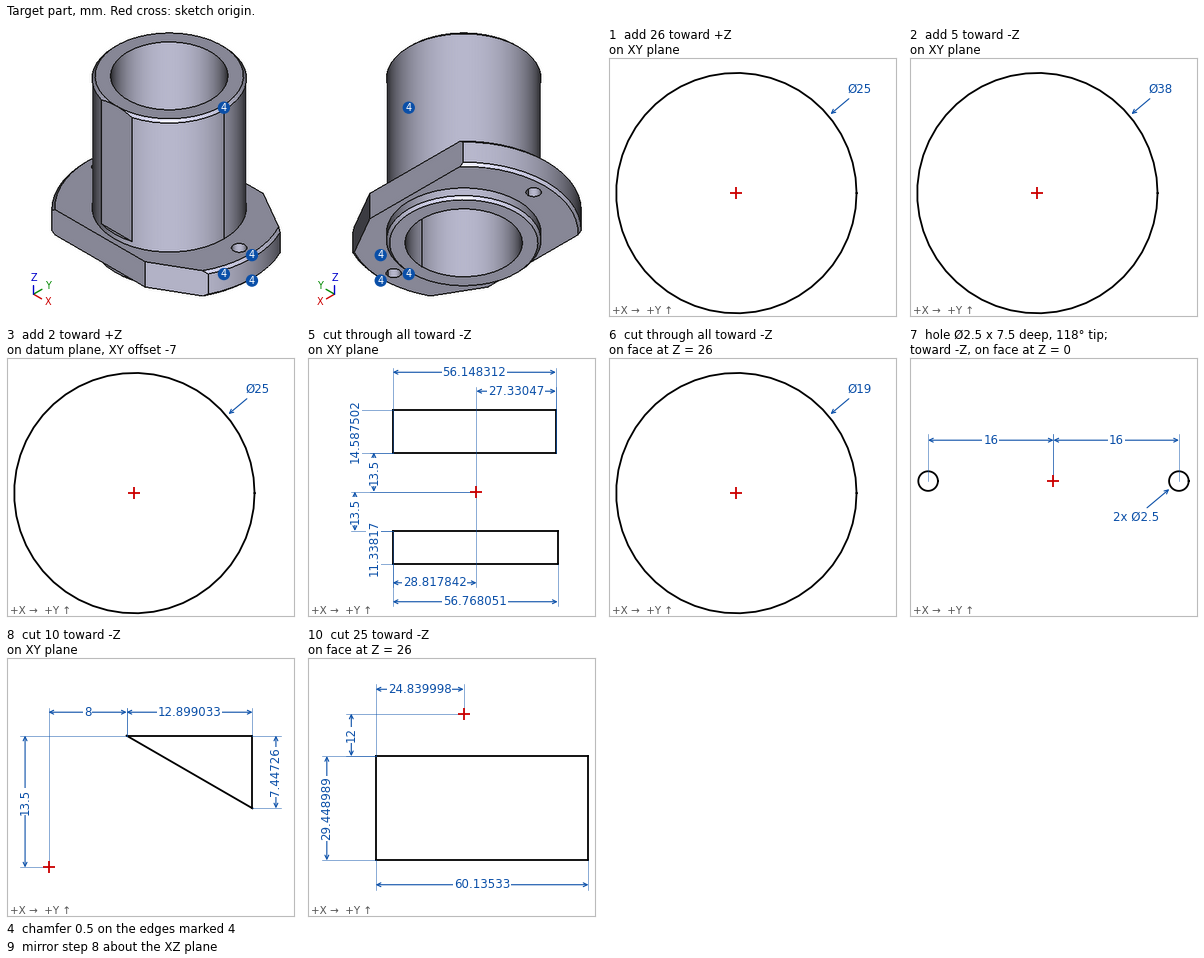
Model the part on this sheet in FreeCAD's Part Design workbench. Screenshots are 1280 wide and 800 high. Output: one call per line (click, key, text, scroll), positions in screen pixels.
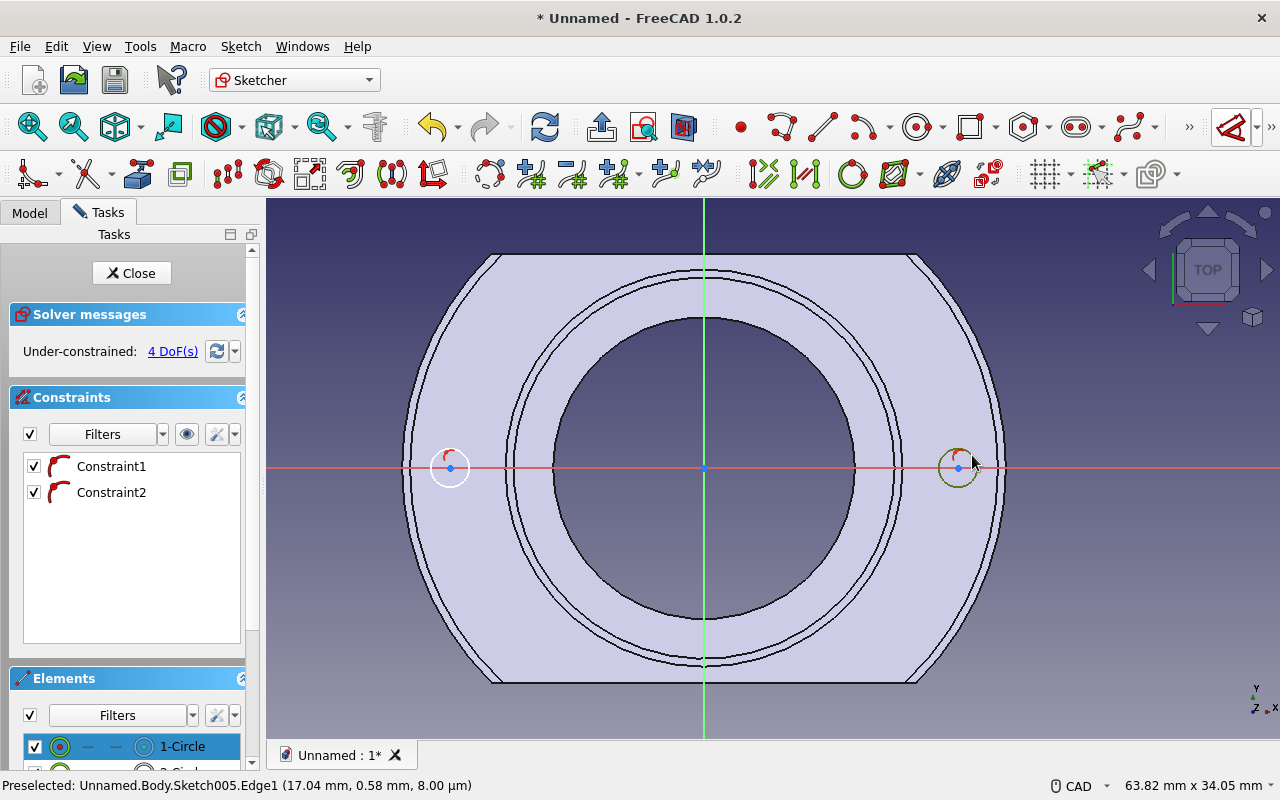
click(464, 455)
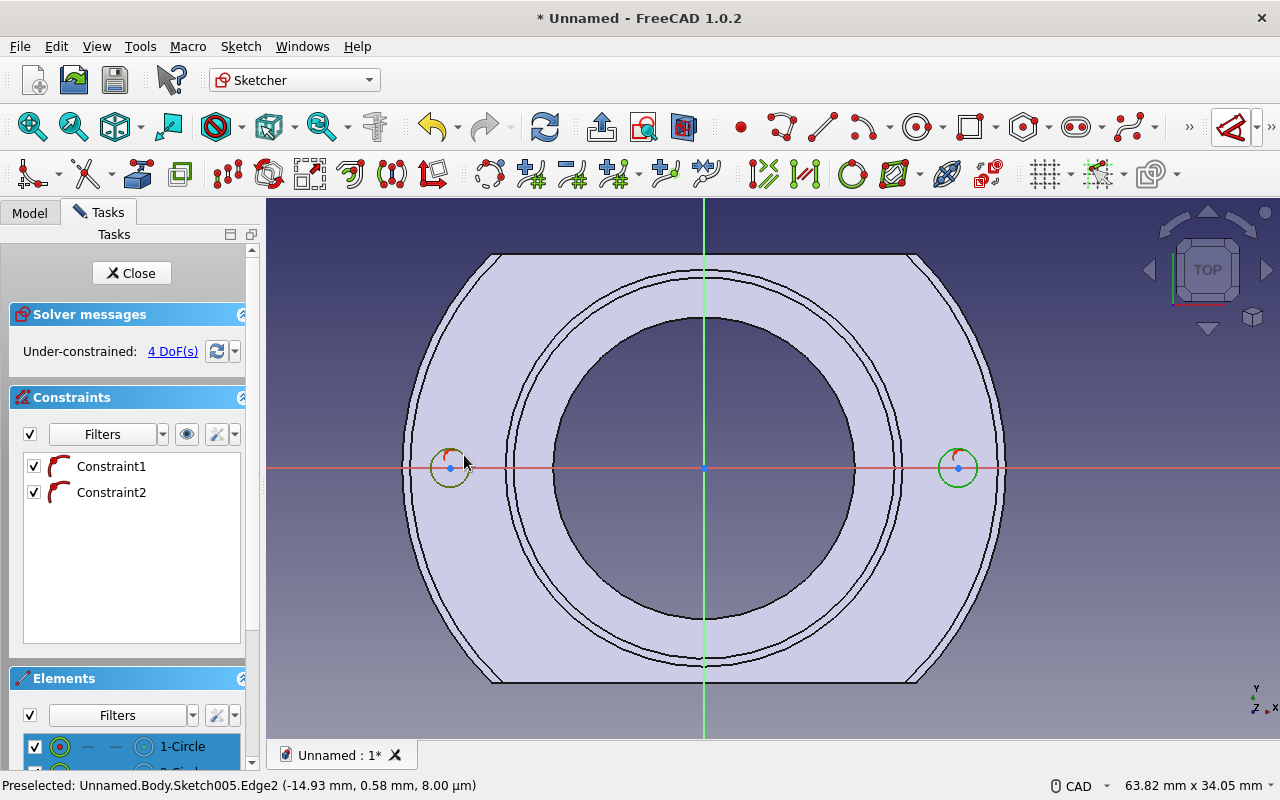
key(e)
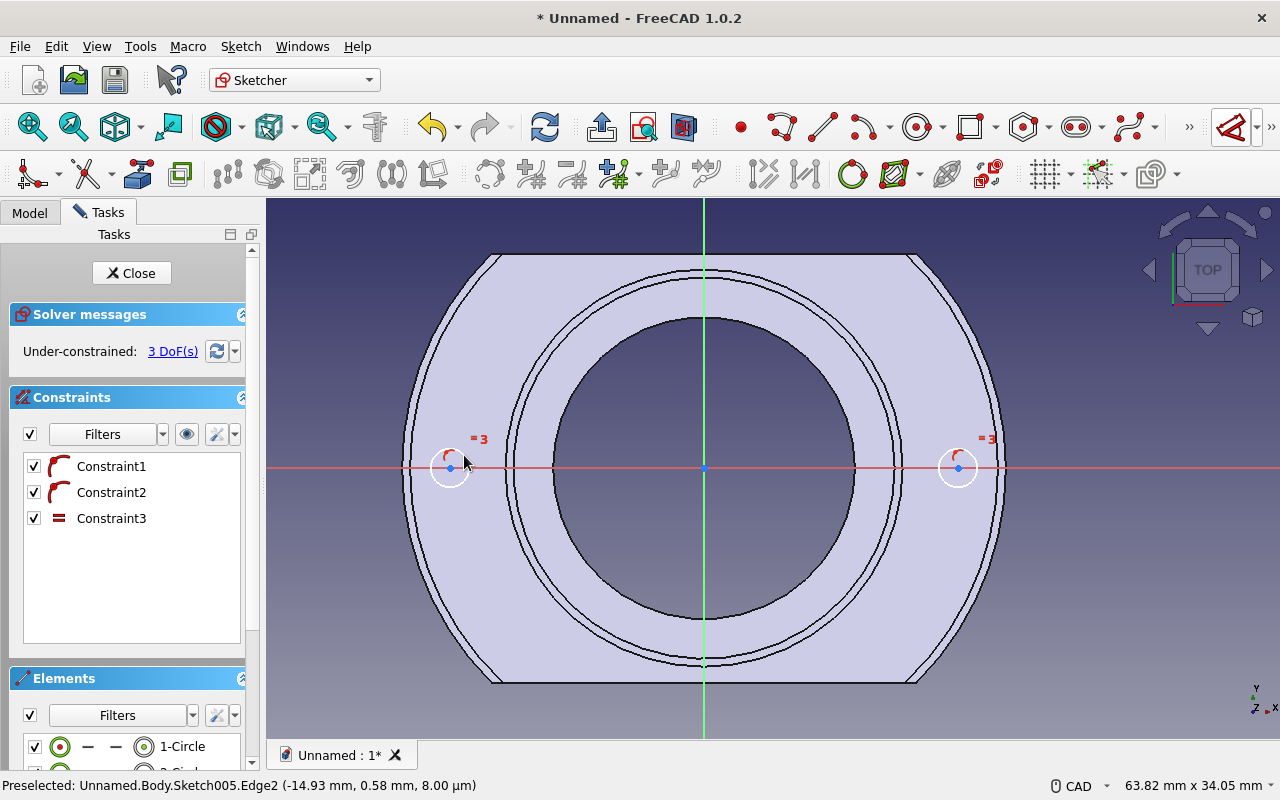
click(972, 455)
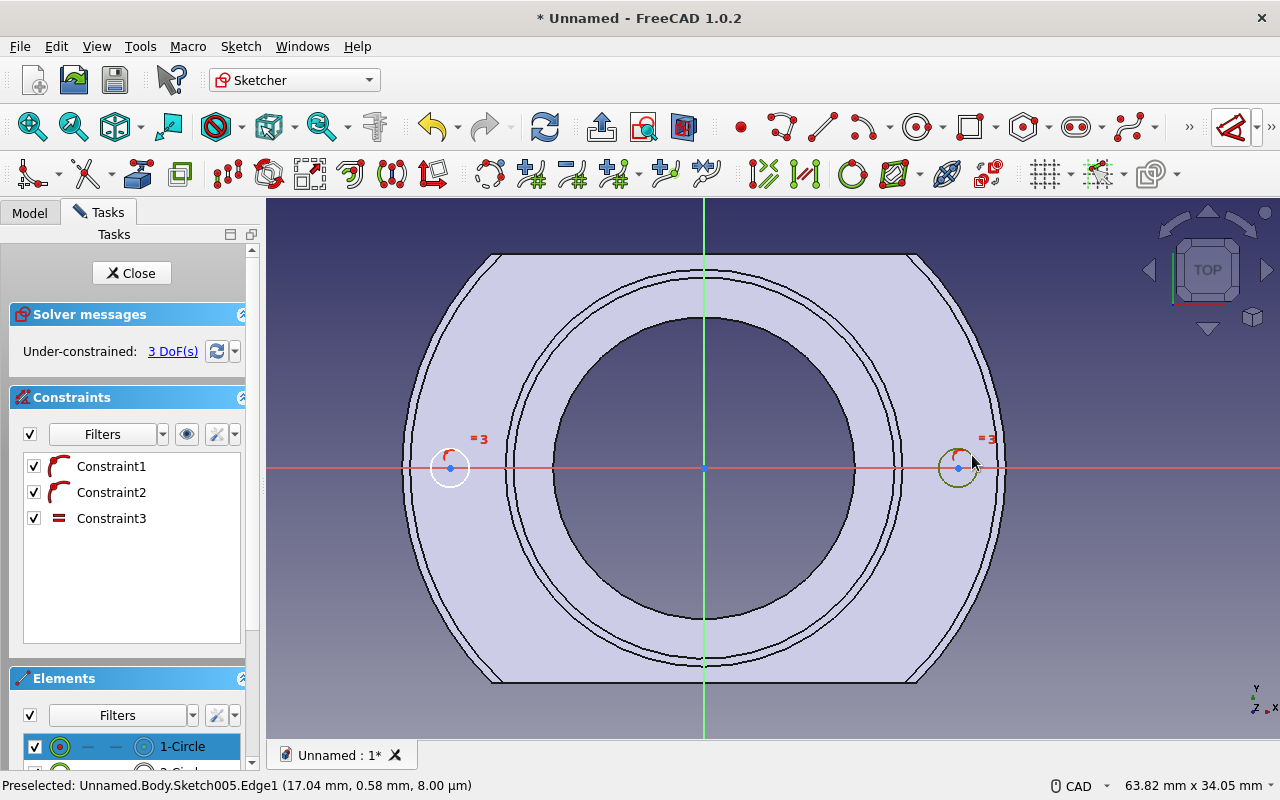
key(k)
key(o)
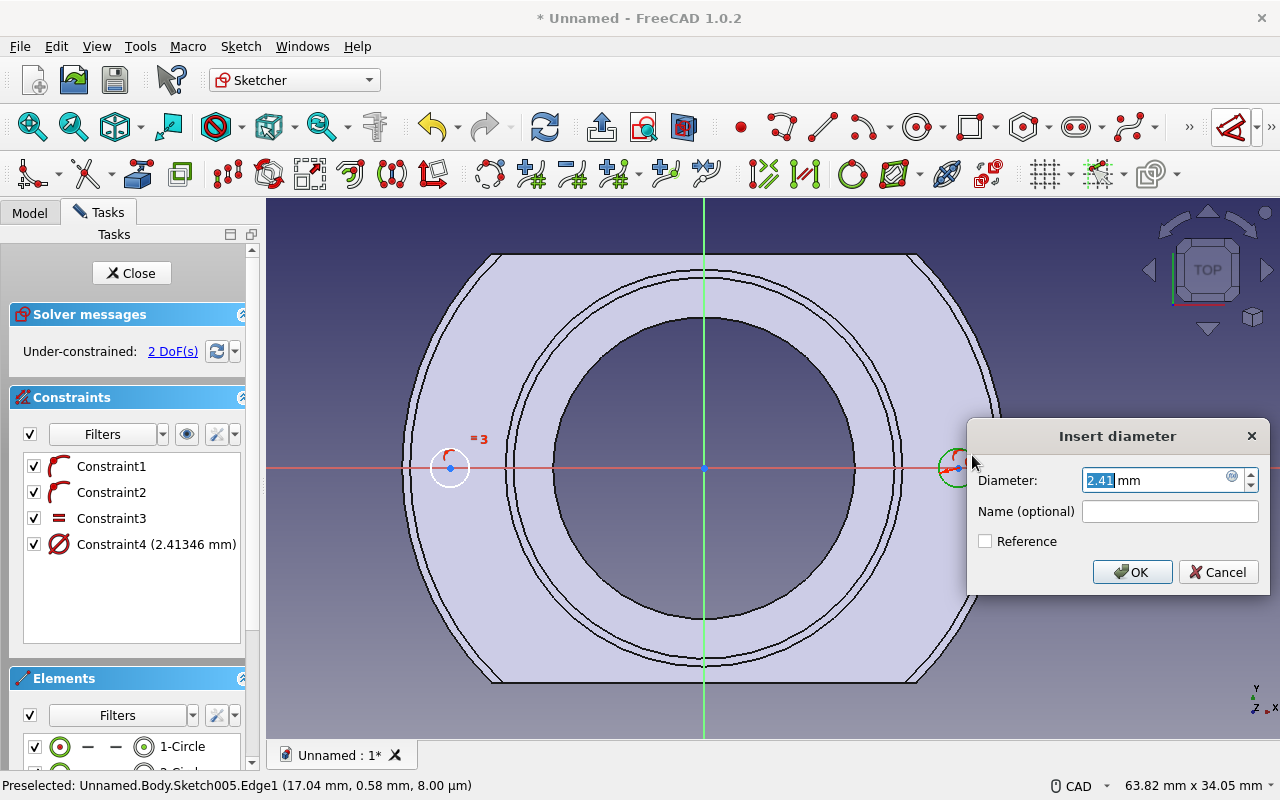
text(2.5)
key(Return)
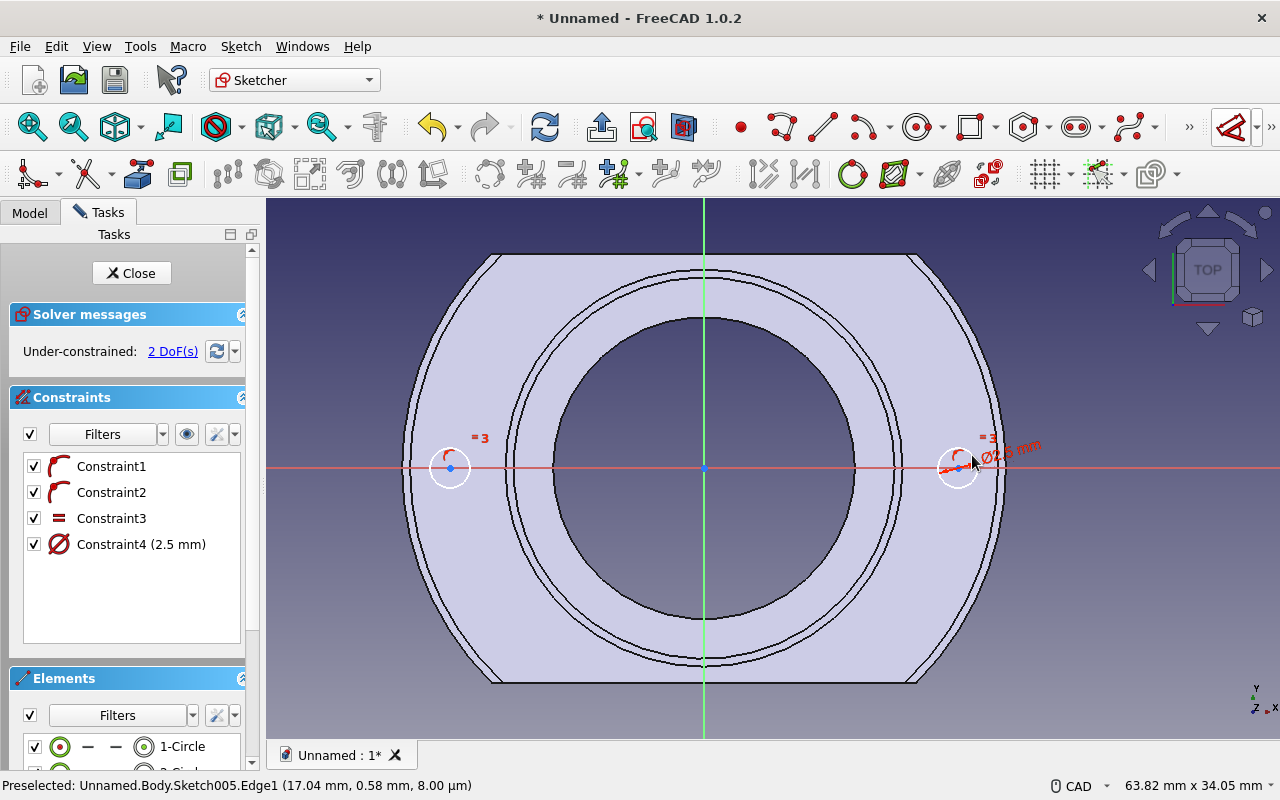
click(958, 468)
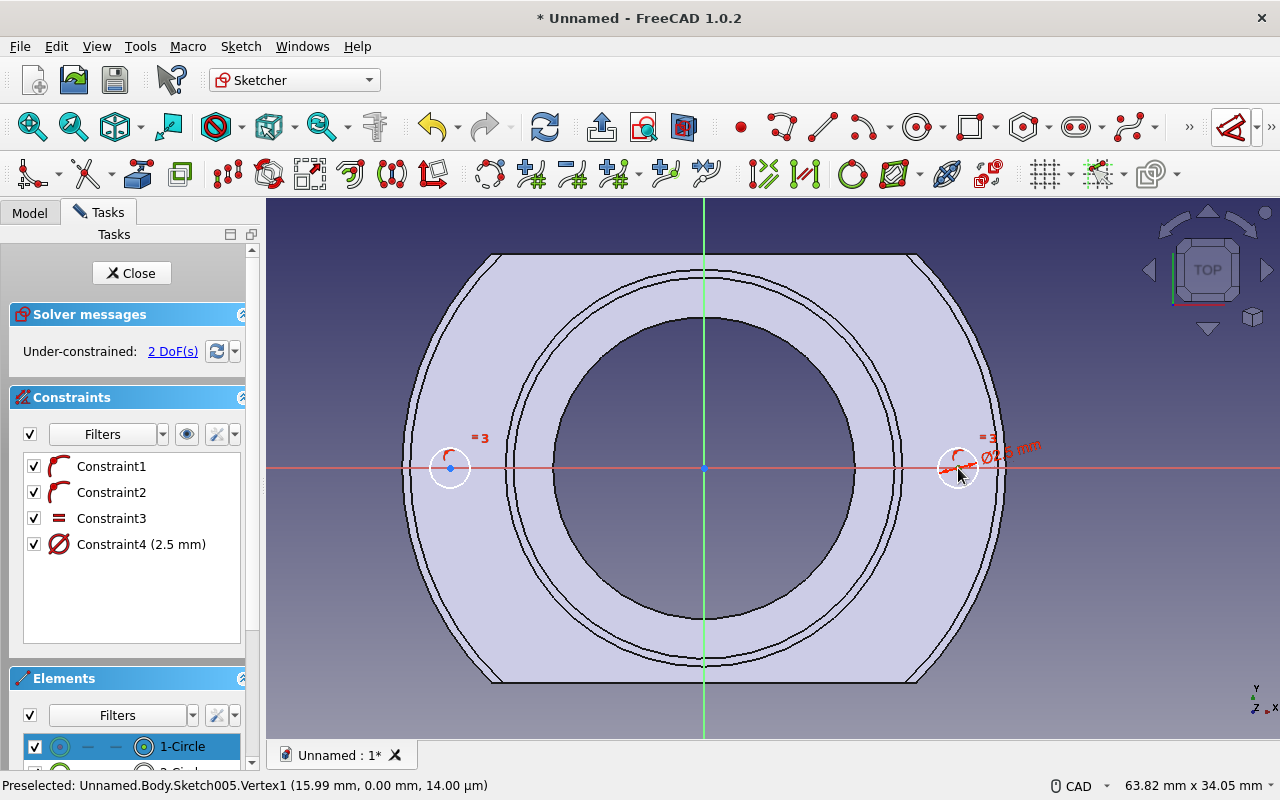
click(1256, 128)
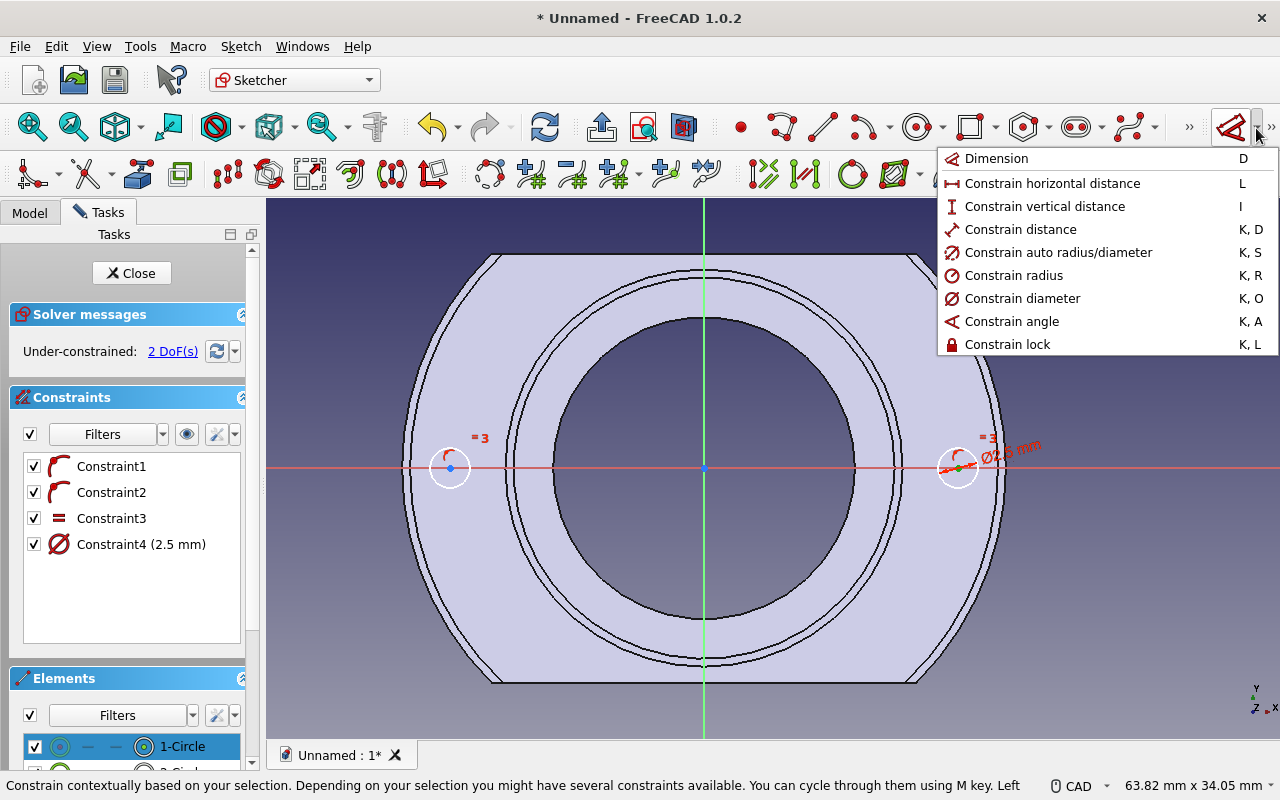
click(1108, 184)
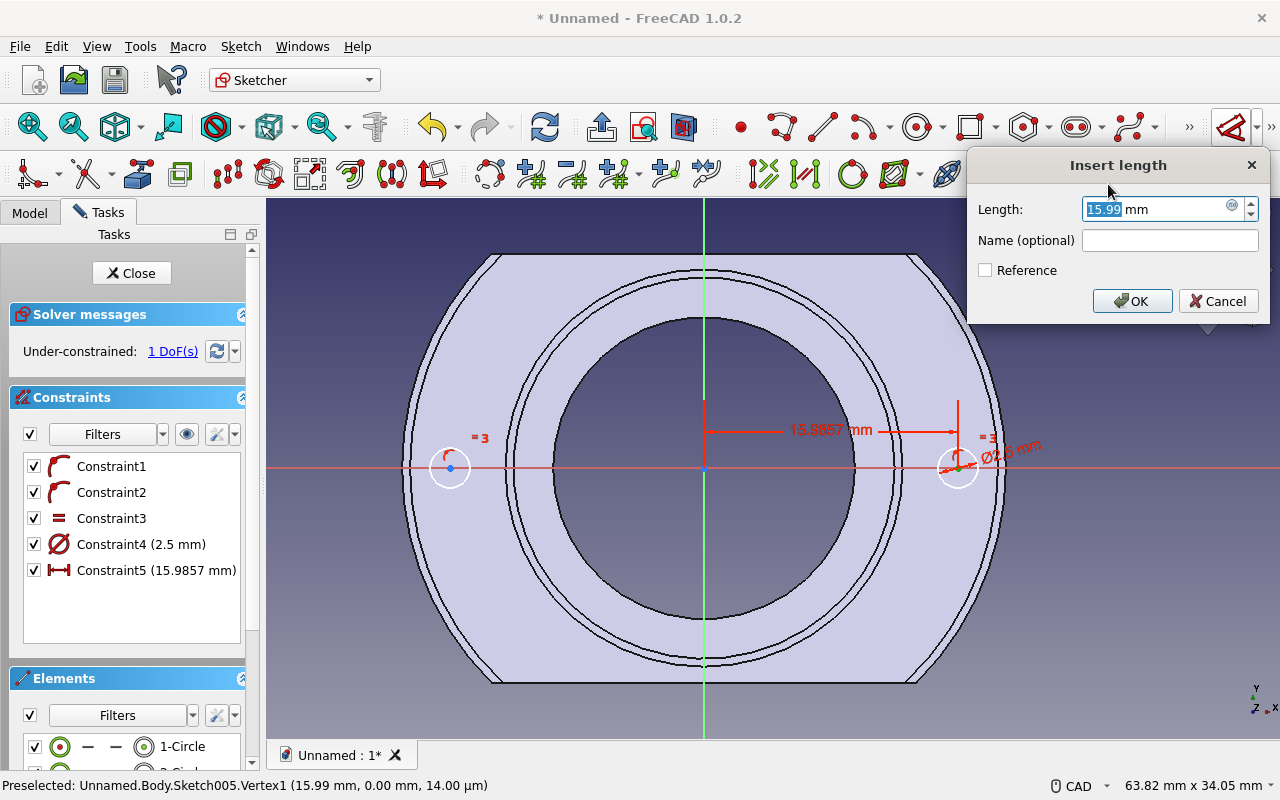
text(16)
key(Return)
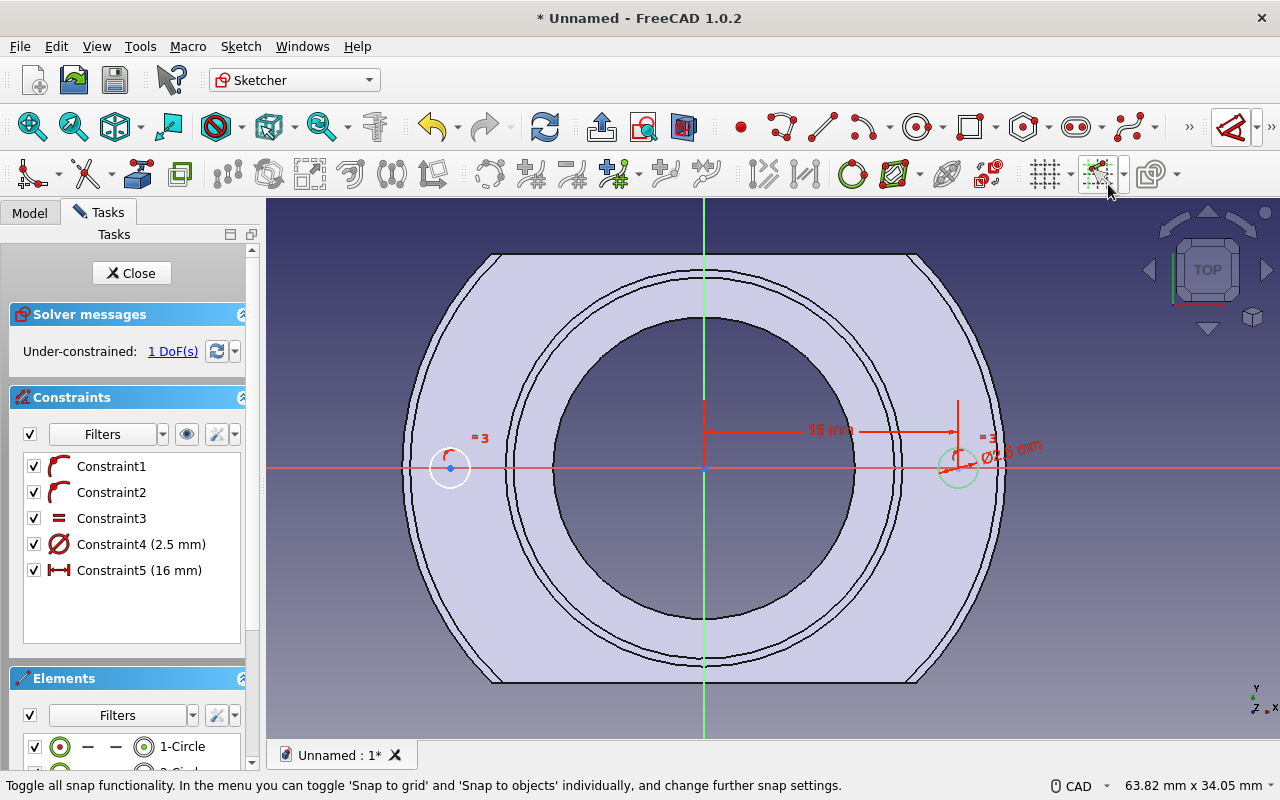
click(450, 468)